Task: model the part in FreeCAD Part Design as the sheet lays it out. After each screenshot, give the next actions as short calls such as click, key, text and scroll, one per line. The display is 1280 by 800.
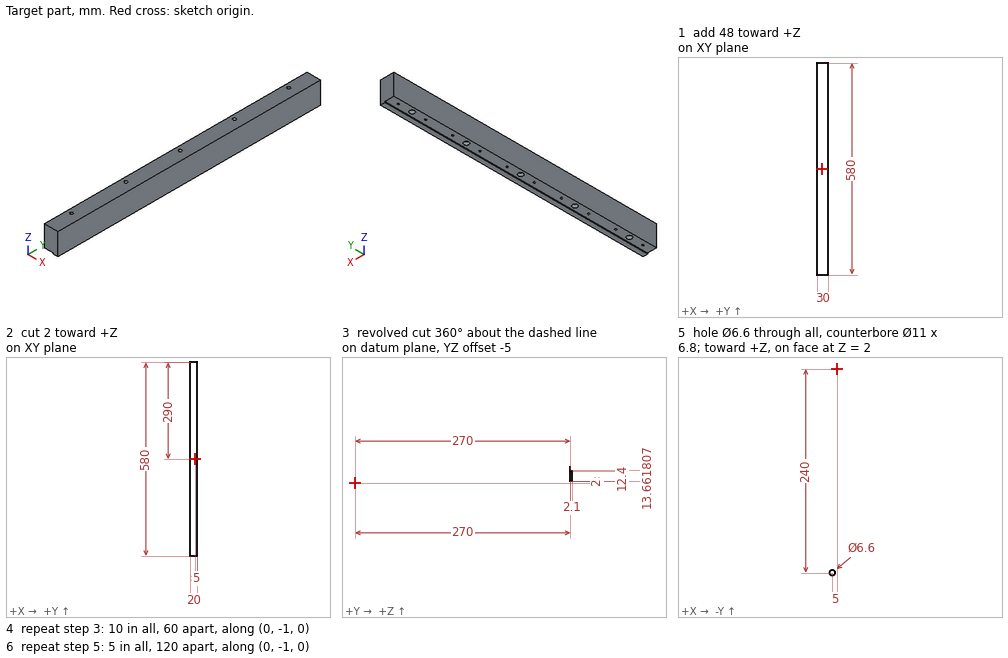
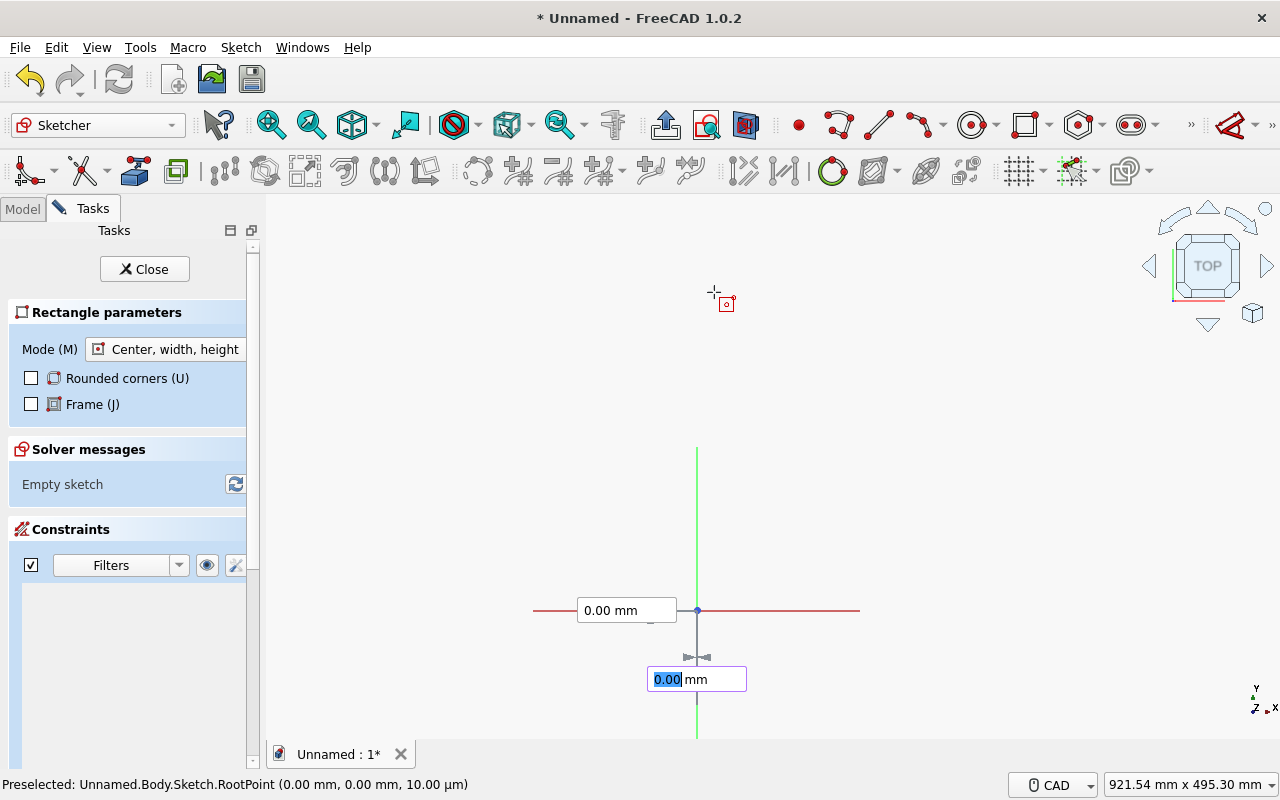
click(714, 292)
key(Escape)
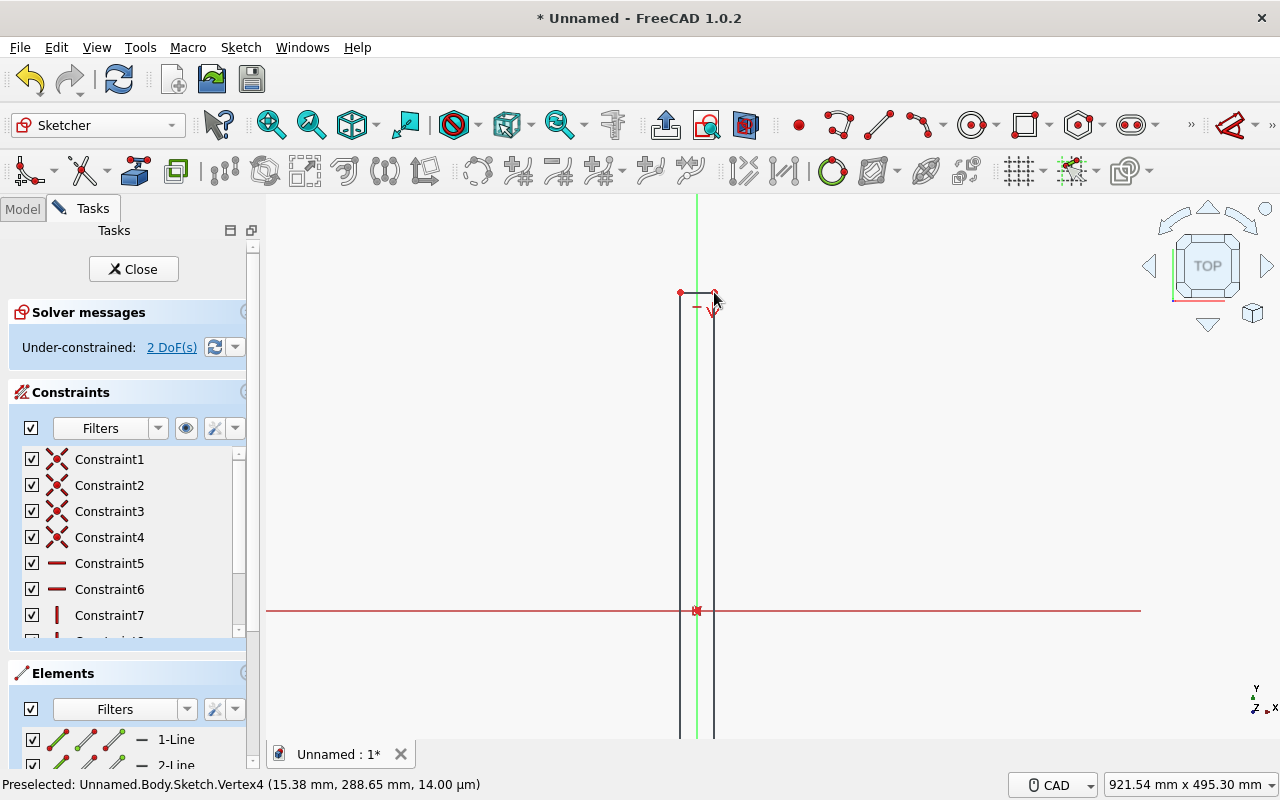
key(d)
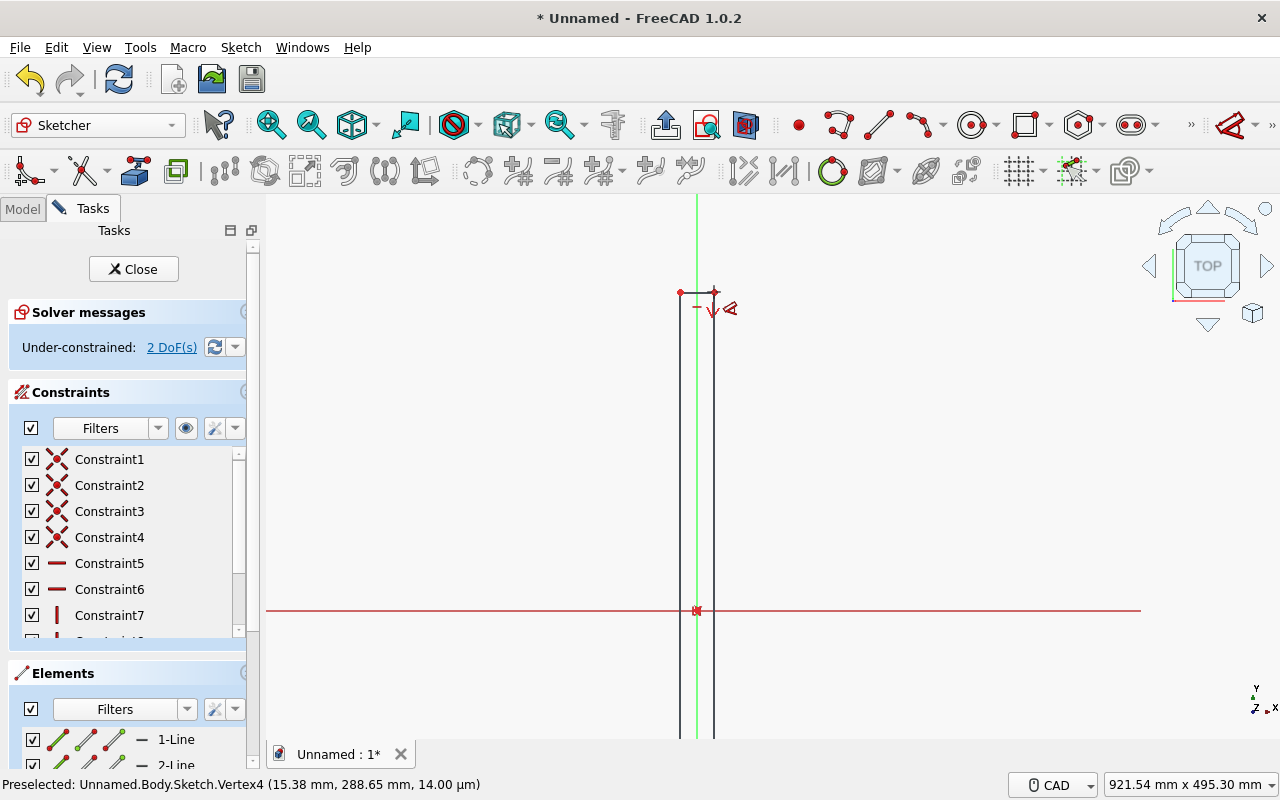
scroll(714, 291, down, 3)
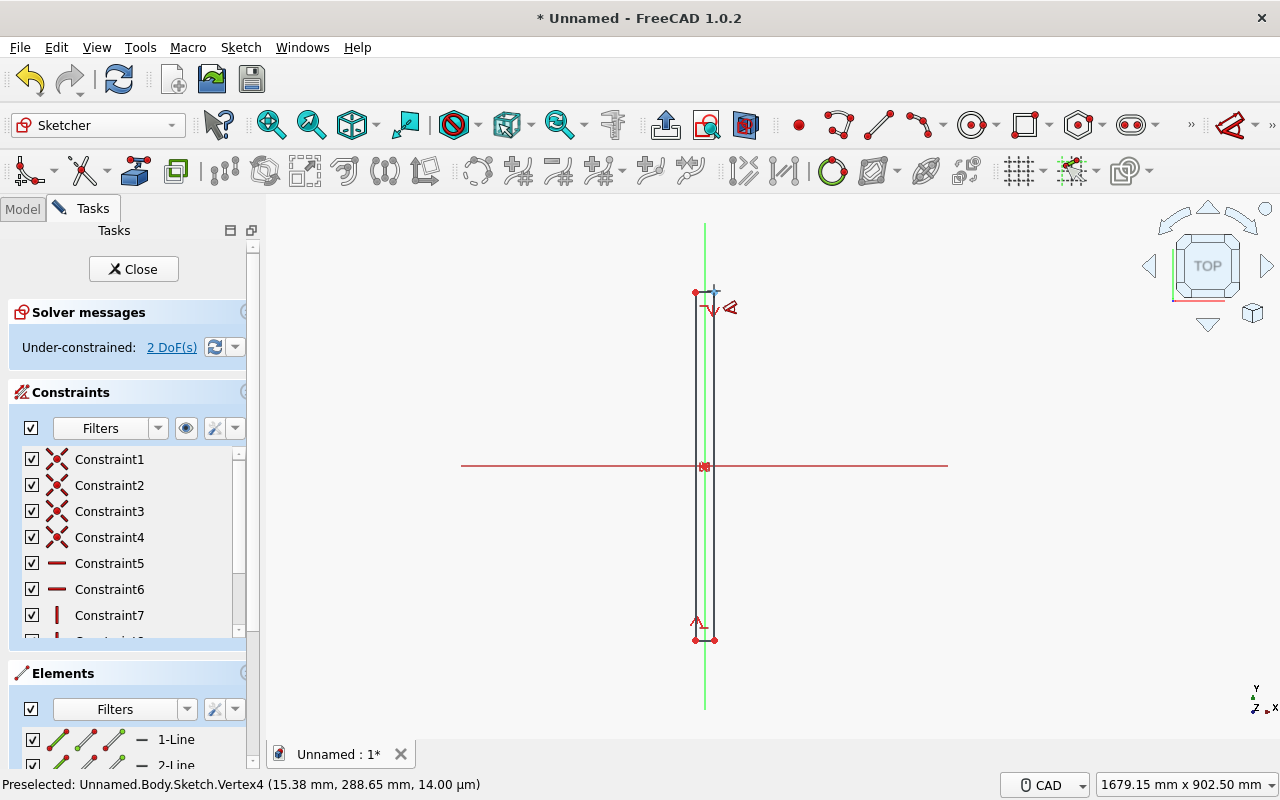
scroll(703, 641, up, 4)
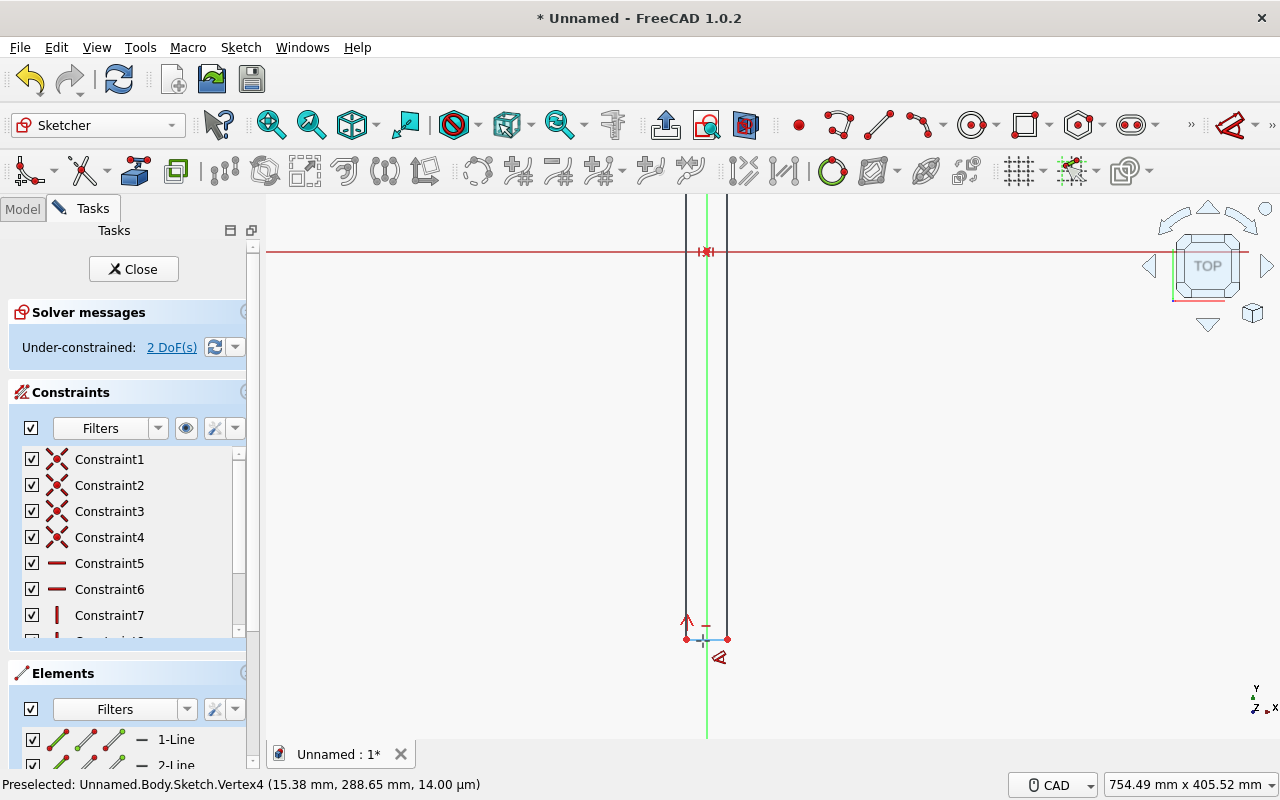
click(703, 640)
click(692, 674)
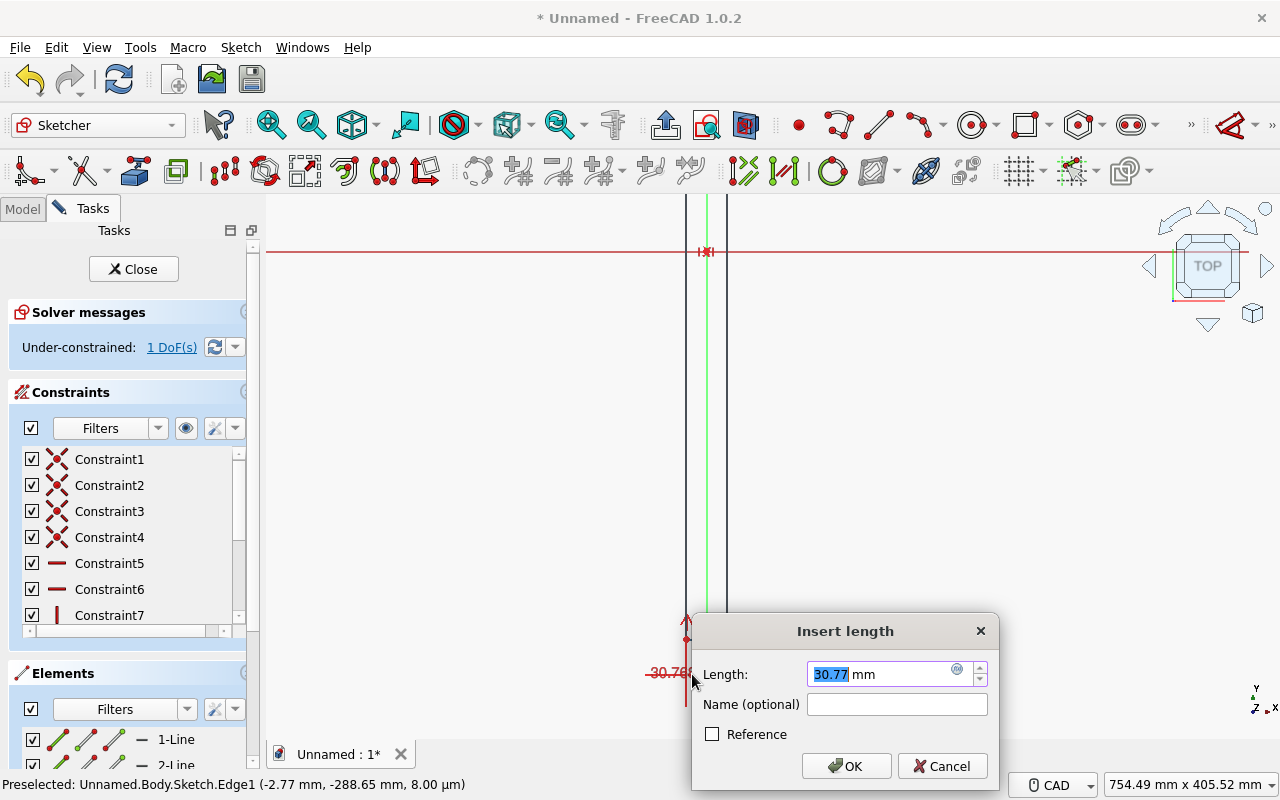
text(30)
key(Return)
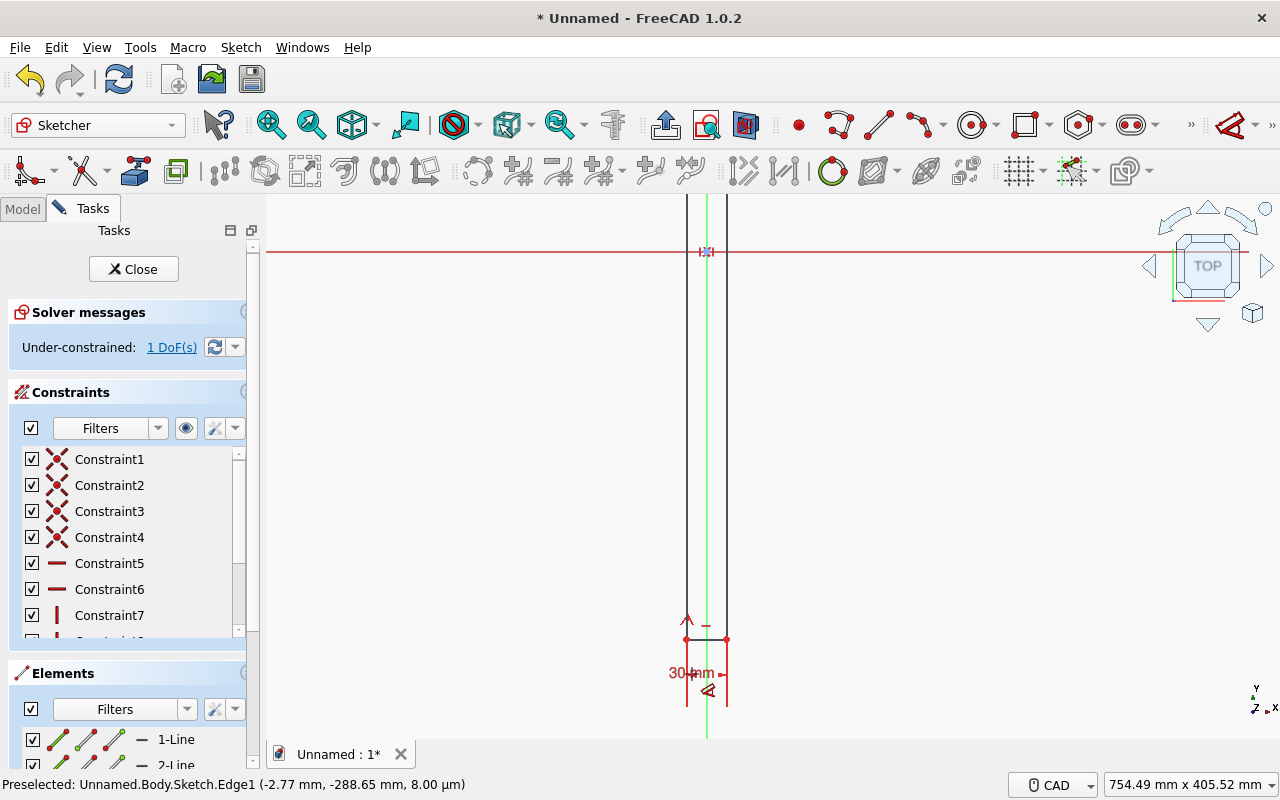
click(727, 407)
click(761, 431)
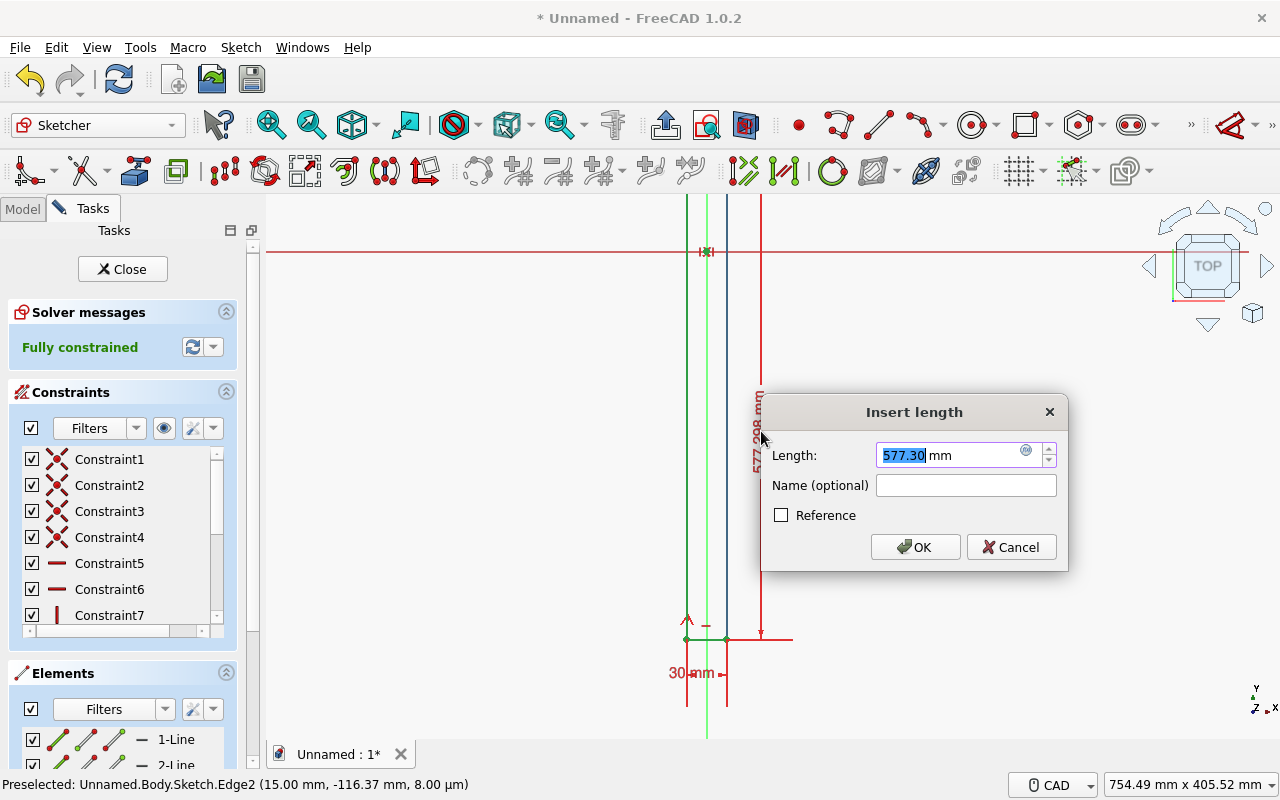
text(580)
key(Return)
key(Escape)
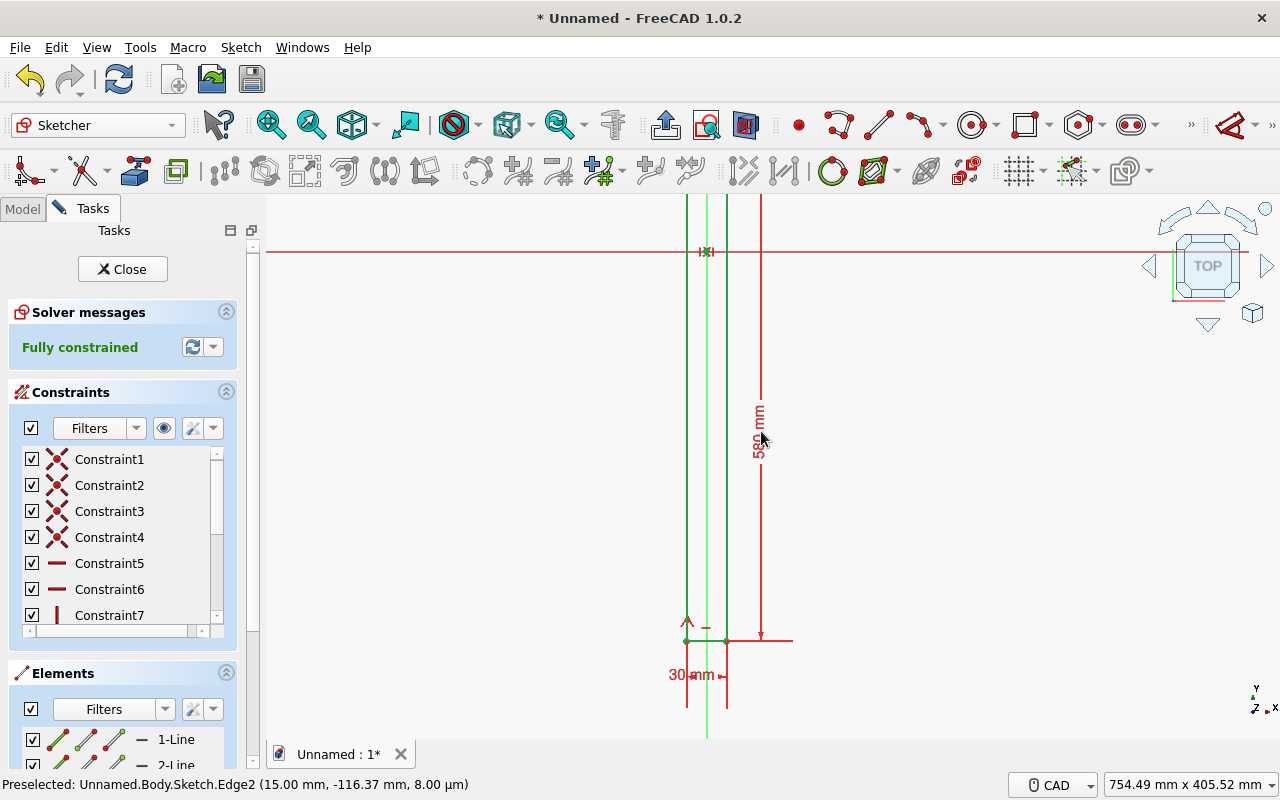
click(123, 269)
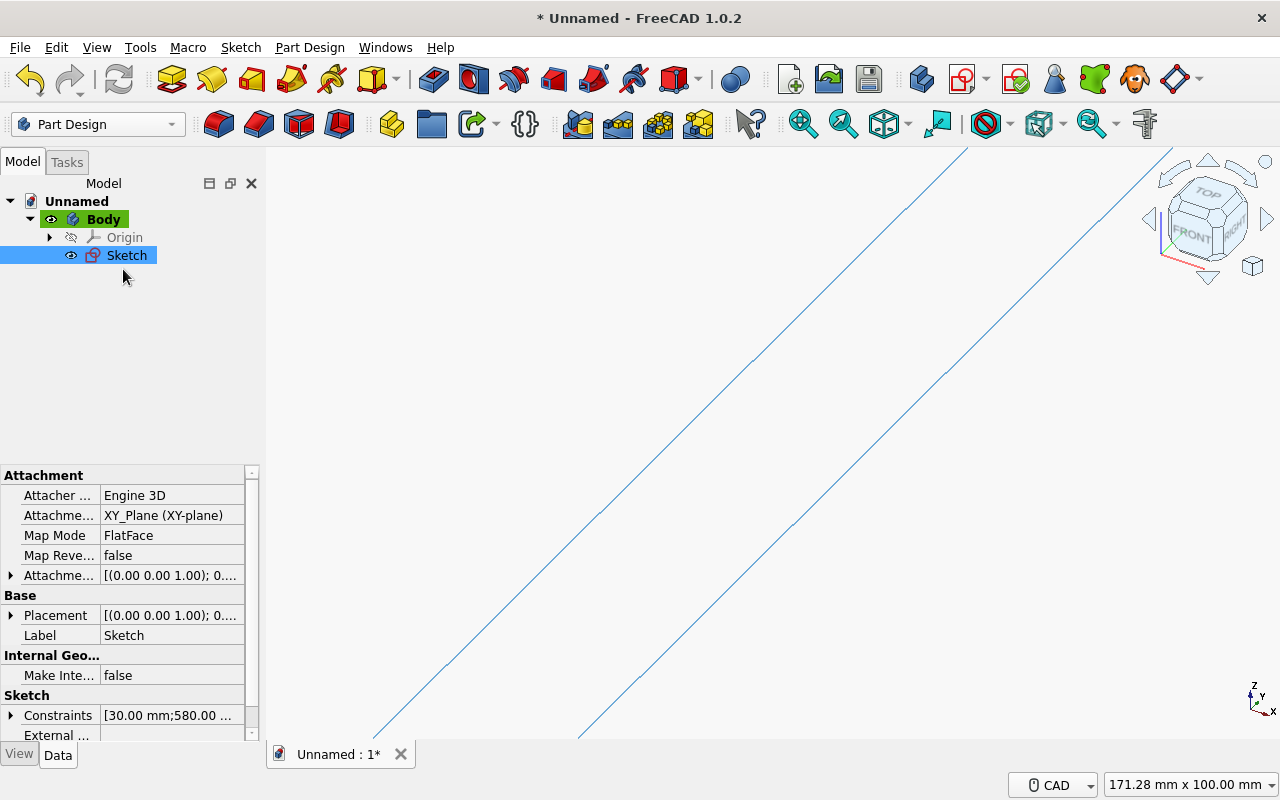
click(172, 80)